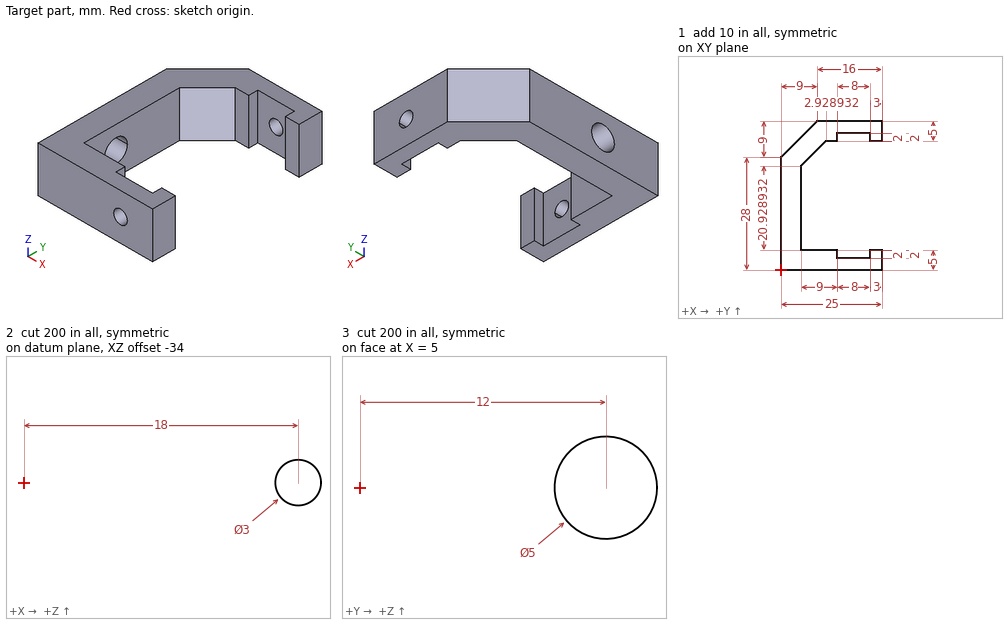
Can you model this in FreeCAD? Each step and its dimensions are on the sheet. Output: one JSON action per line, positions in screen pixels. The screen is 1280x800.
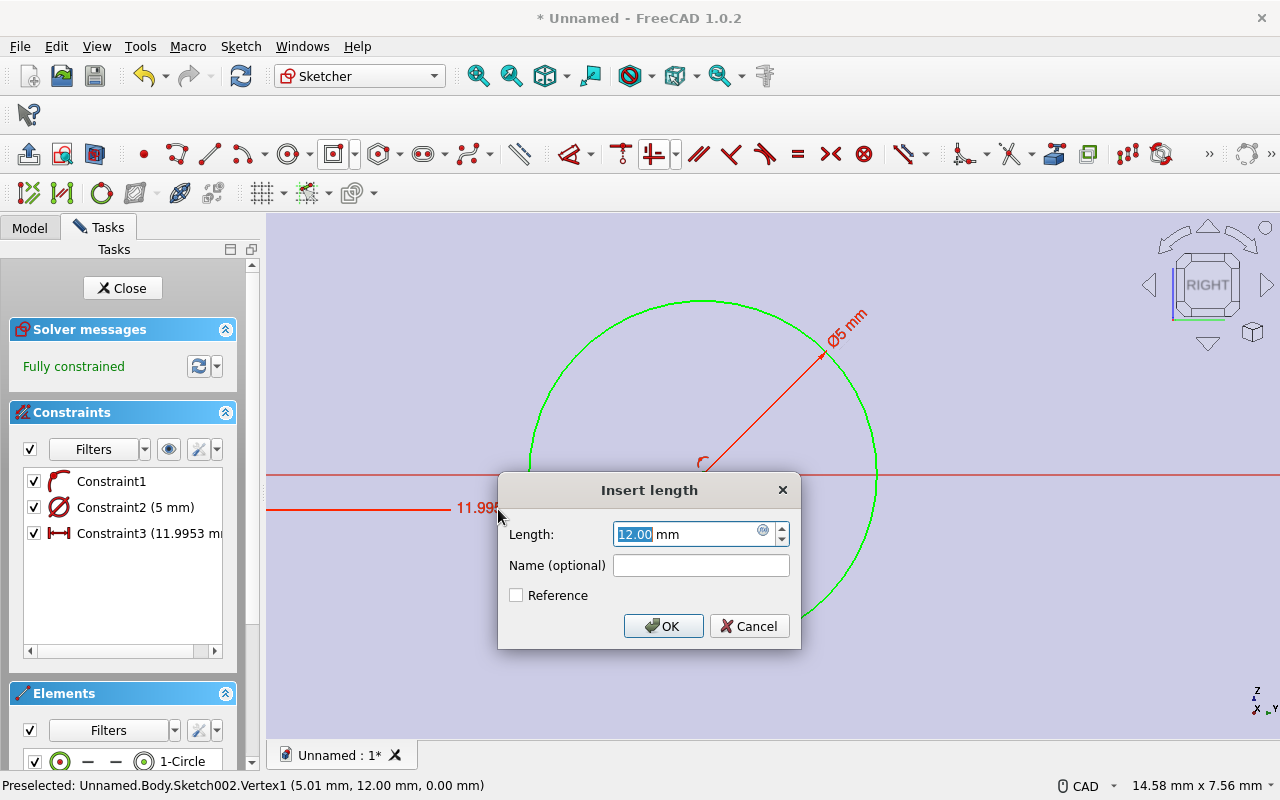
{"action": "type", "text": "12"}
{"action": "key", "text": "Return"}
{"action": "key", "text": "Escape"}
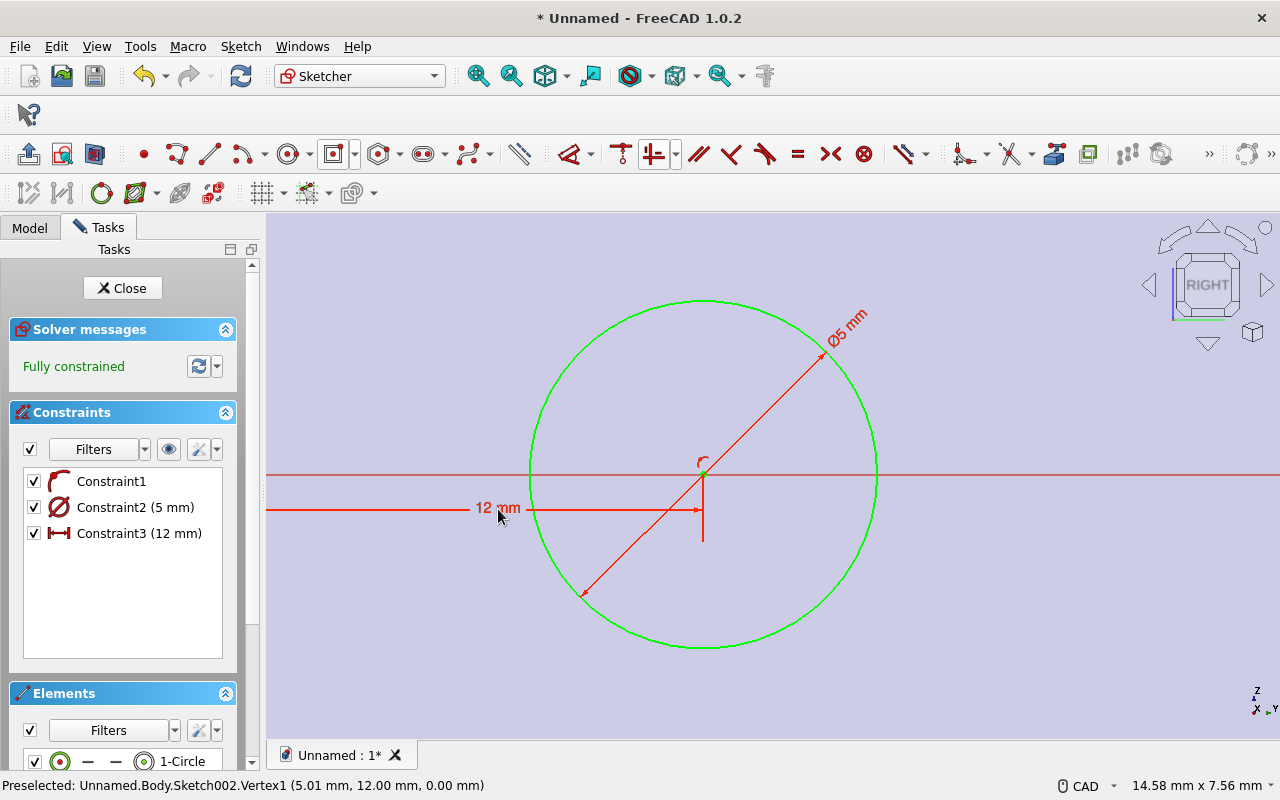
{"action": "left_click", "coordinate": [123, 288]}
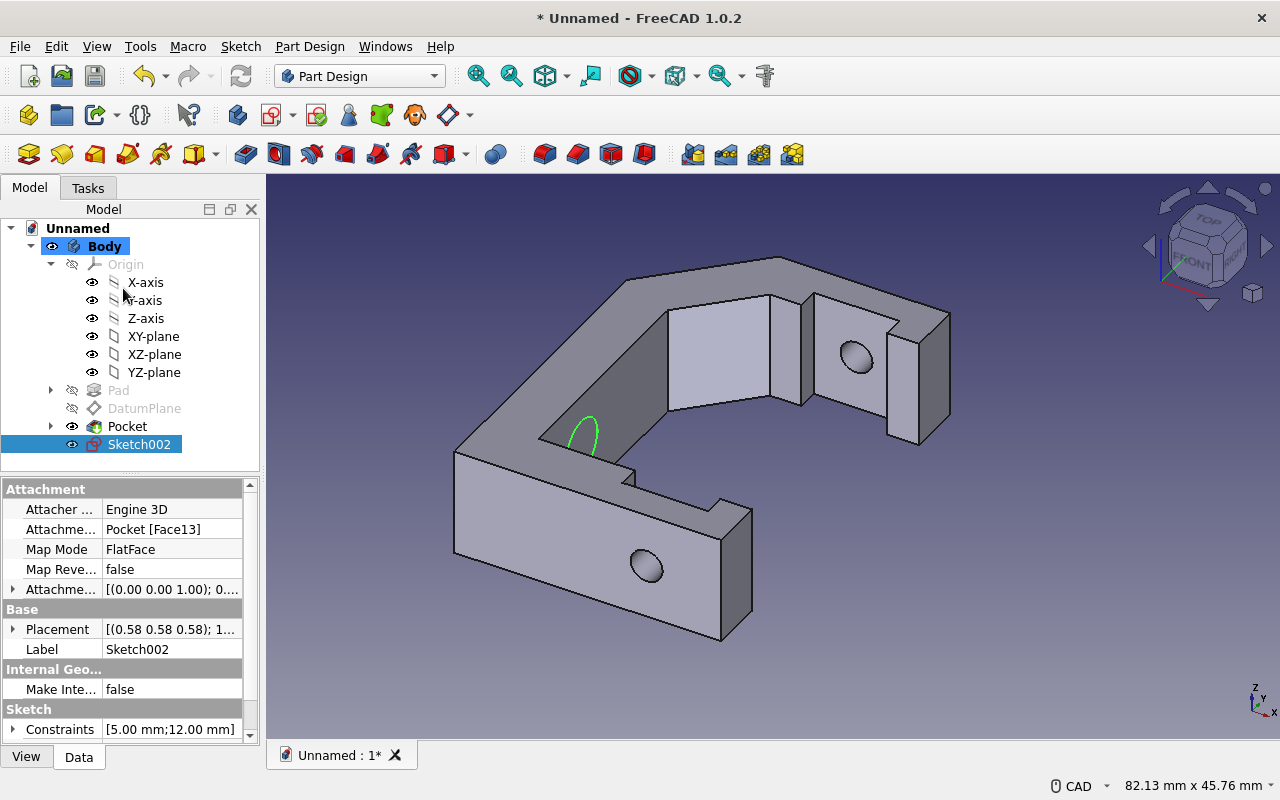
{"action": "left_click", "coordinate": [246, 154]}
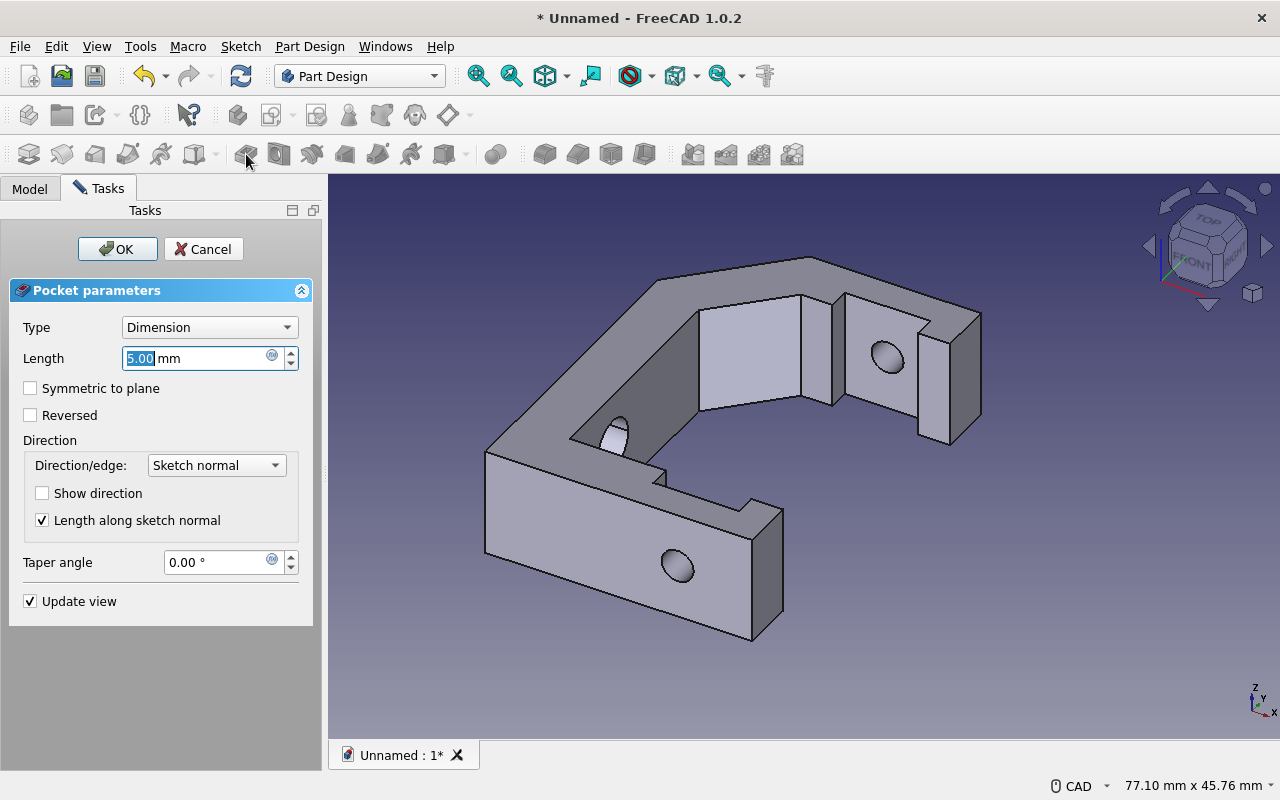
{"action": "type", "text": "200"}
{"action": "key", "text": "Tab"}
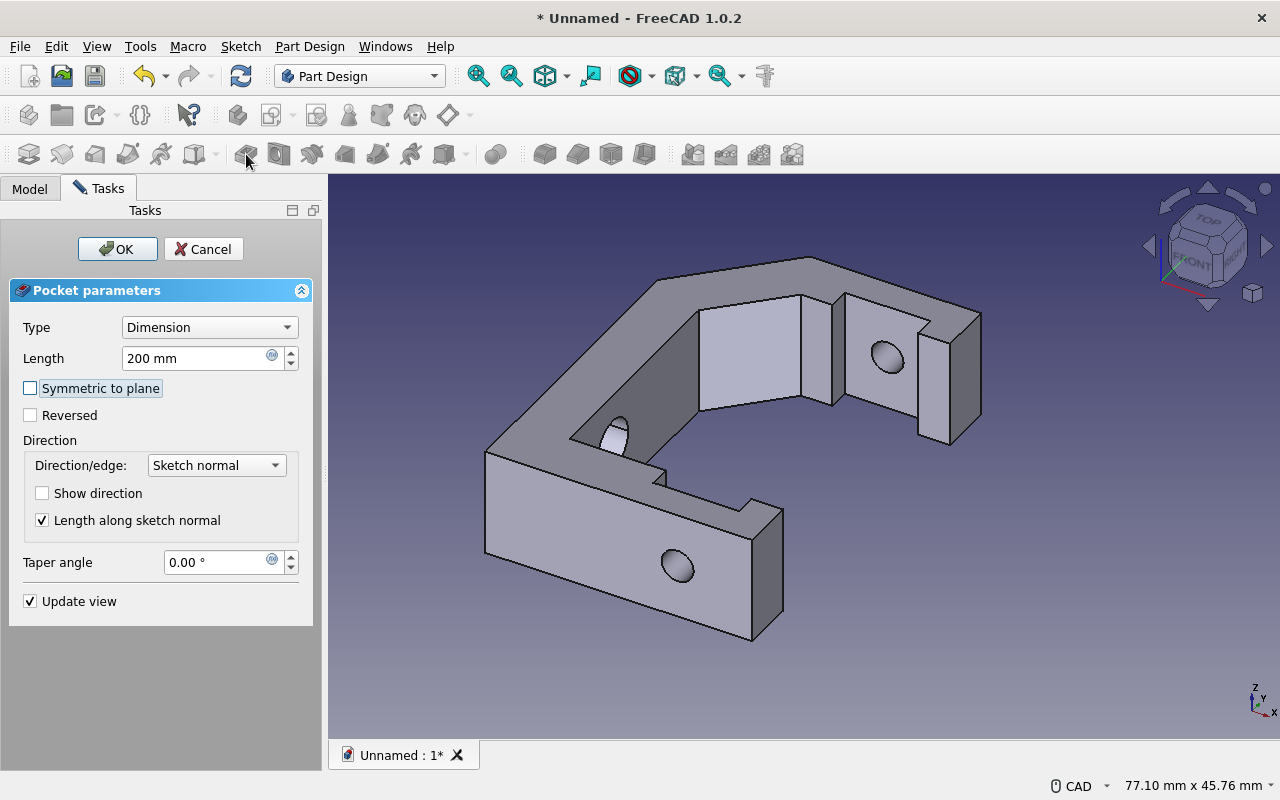
{"action": "left_click", "coordinate": [31, 388]}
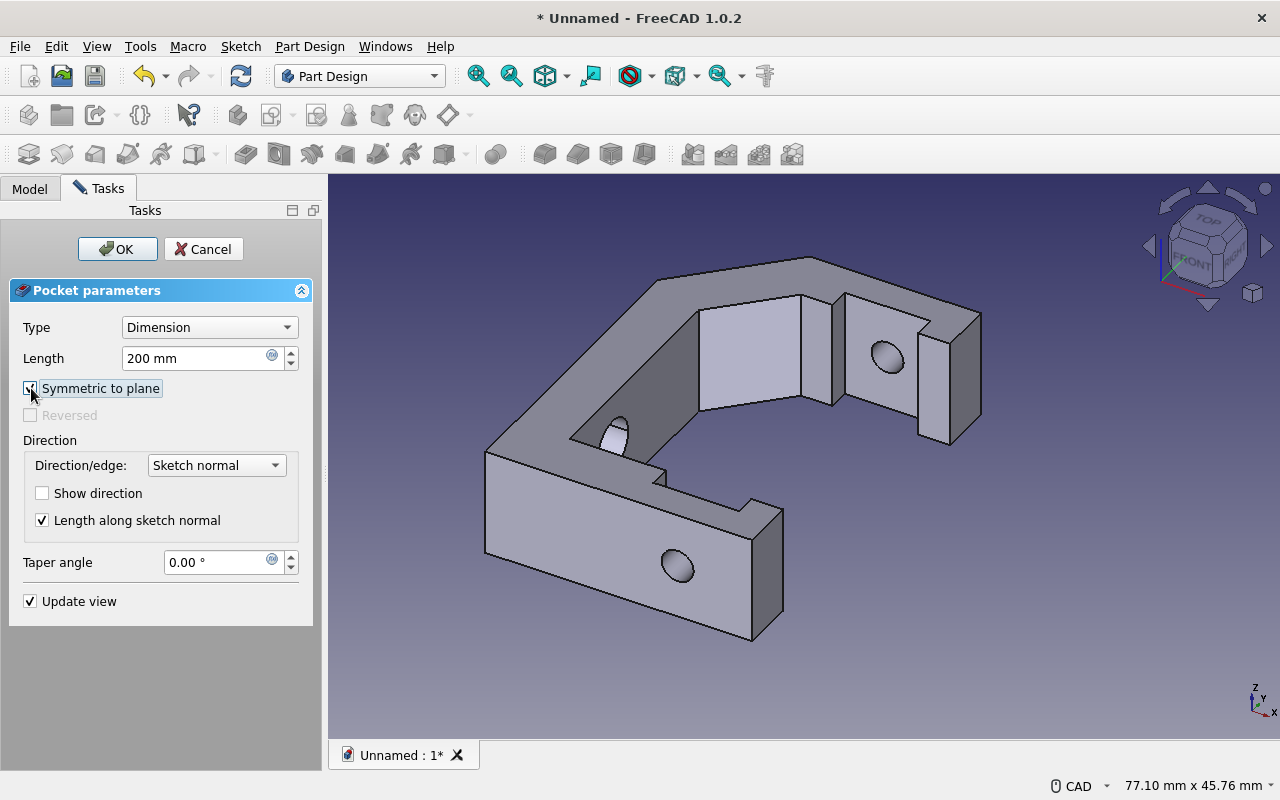
{"action": "left_click", "coordinate": [118, 249]}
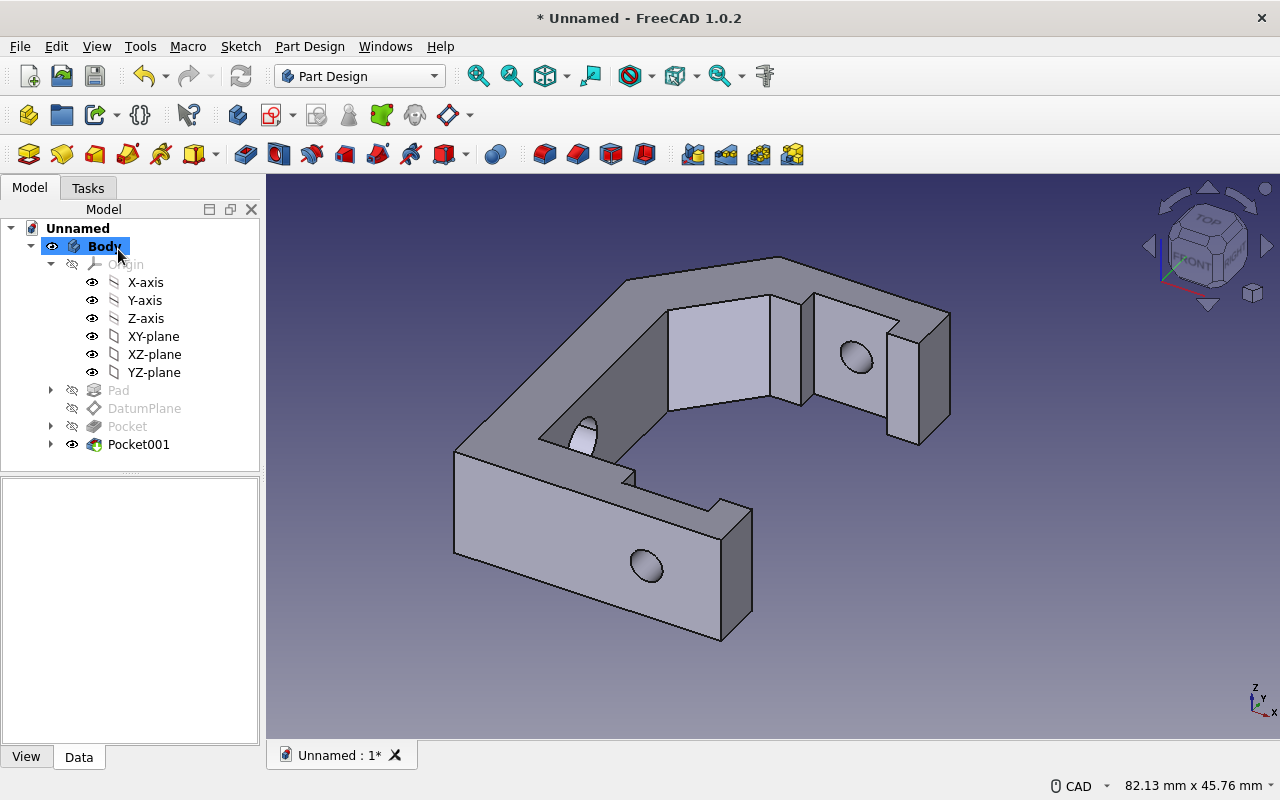
{"action": "key", "text": "0"}